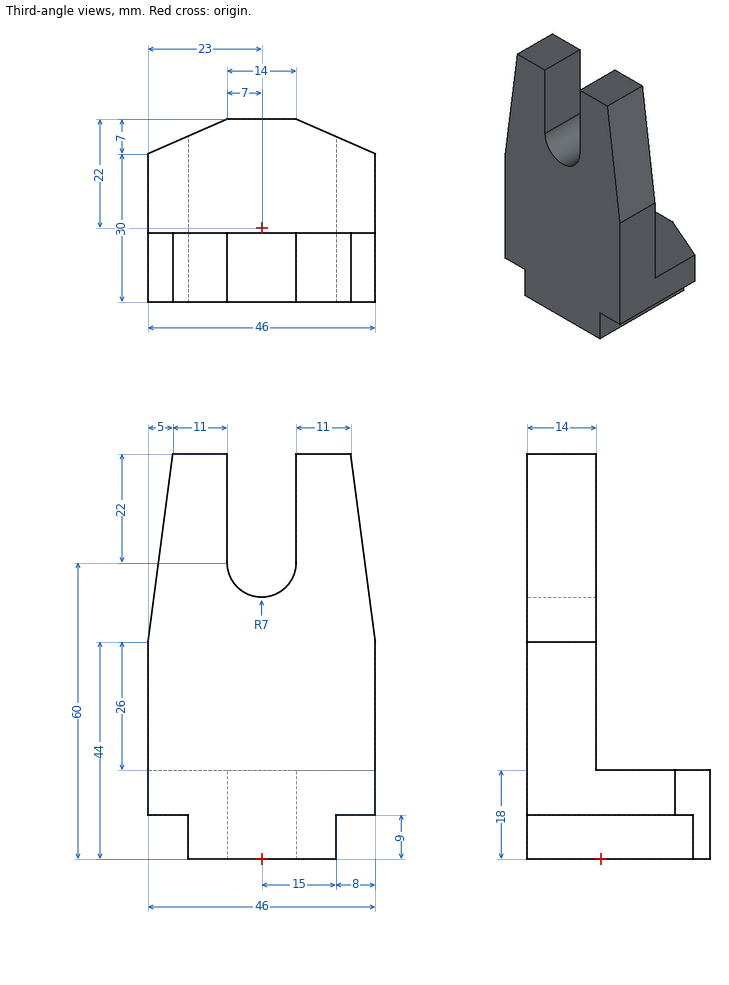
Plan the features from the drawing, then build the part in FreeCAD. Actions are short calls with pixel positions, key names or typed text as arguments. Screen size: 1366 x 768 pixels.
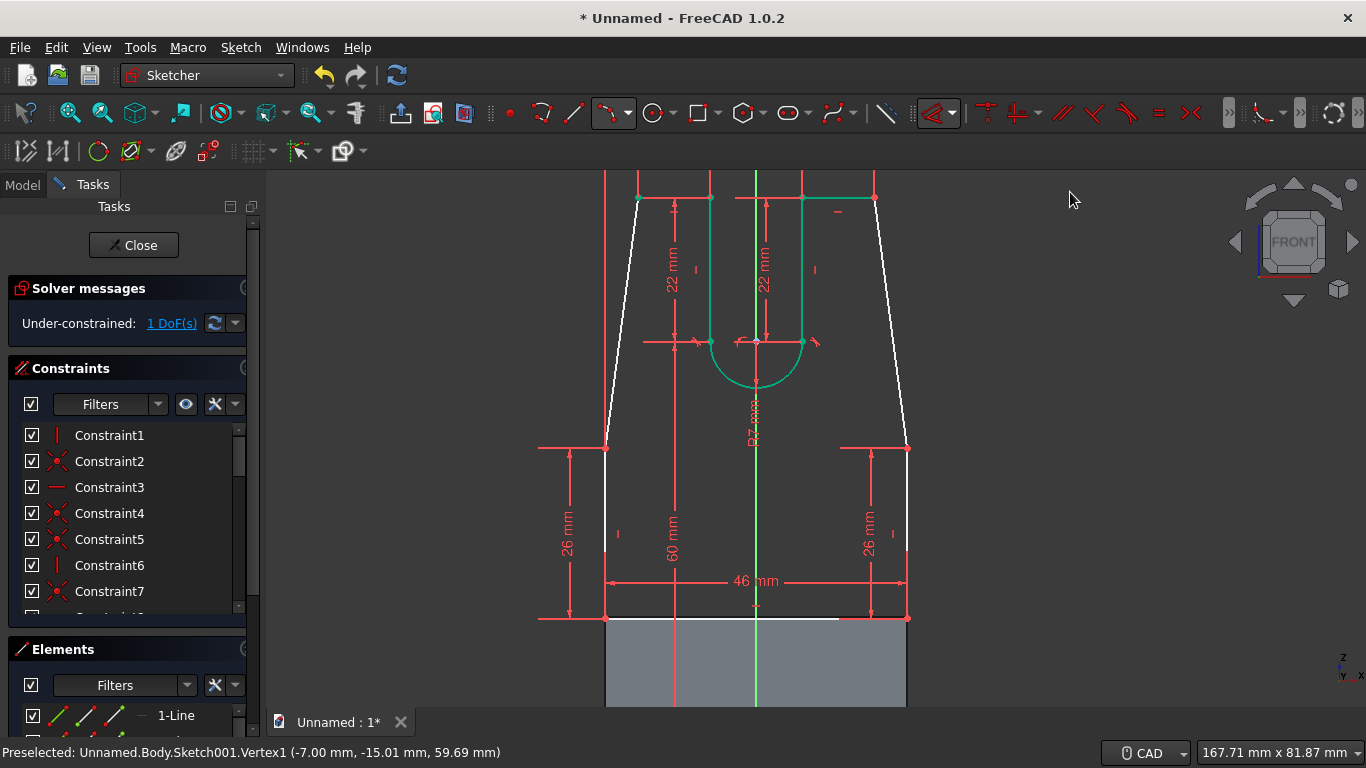
click(605, 448)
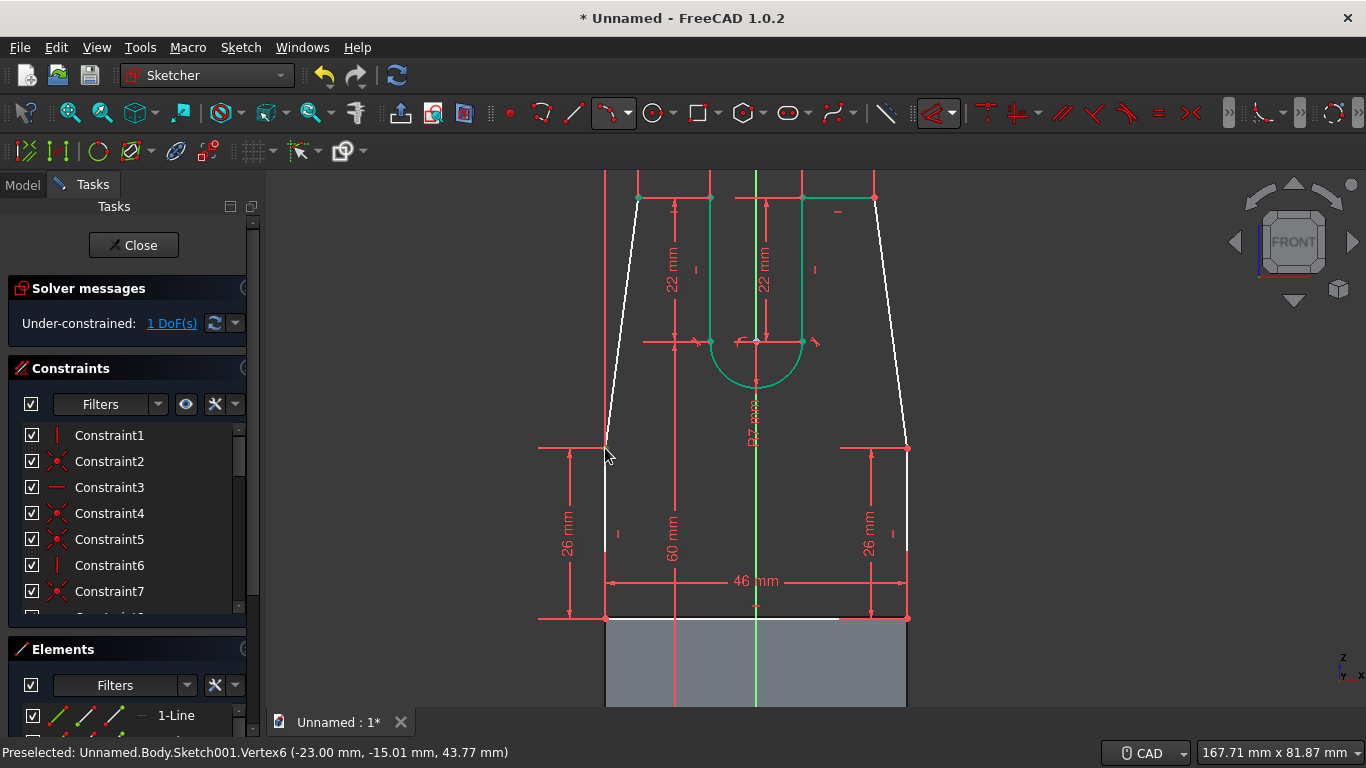
click(954, 114)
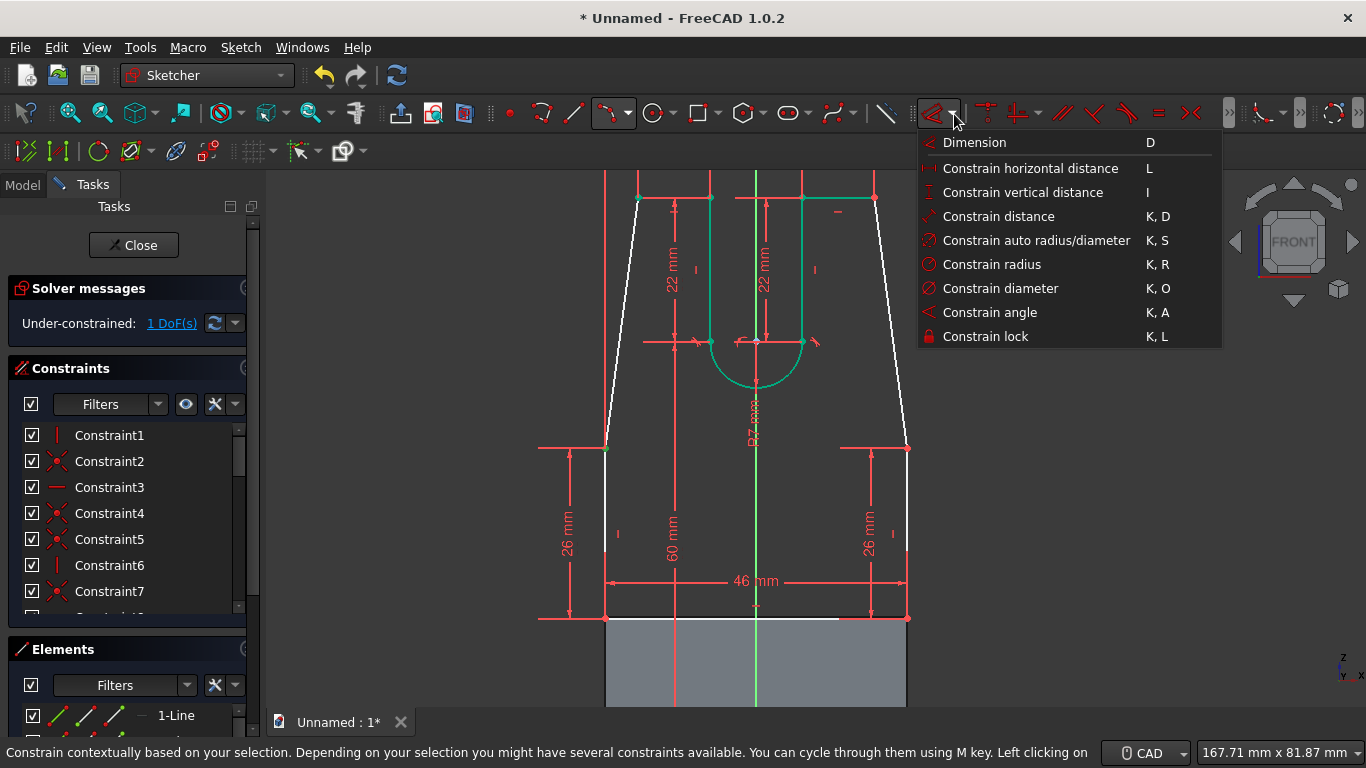
click(1070, 192)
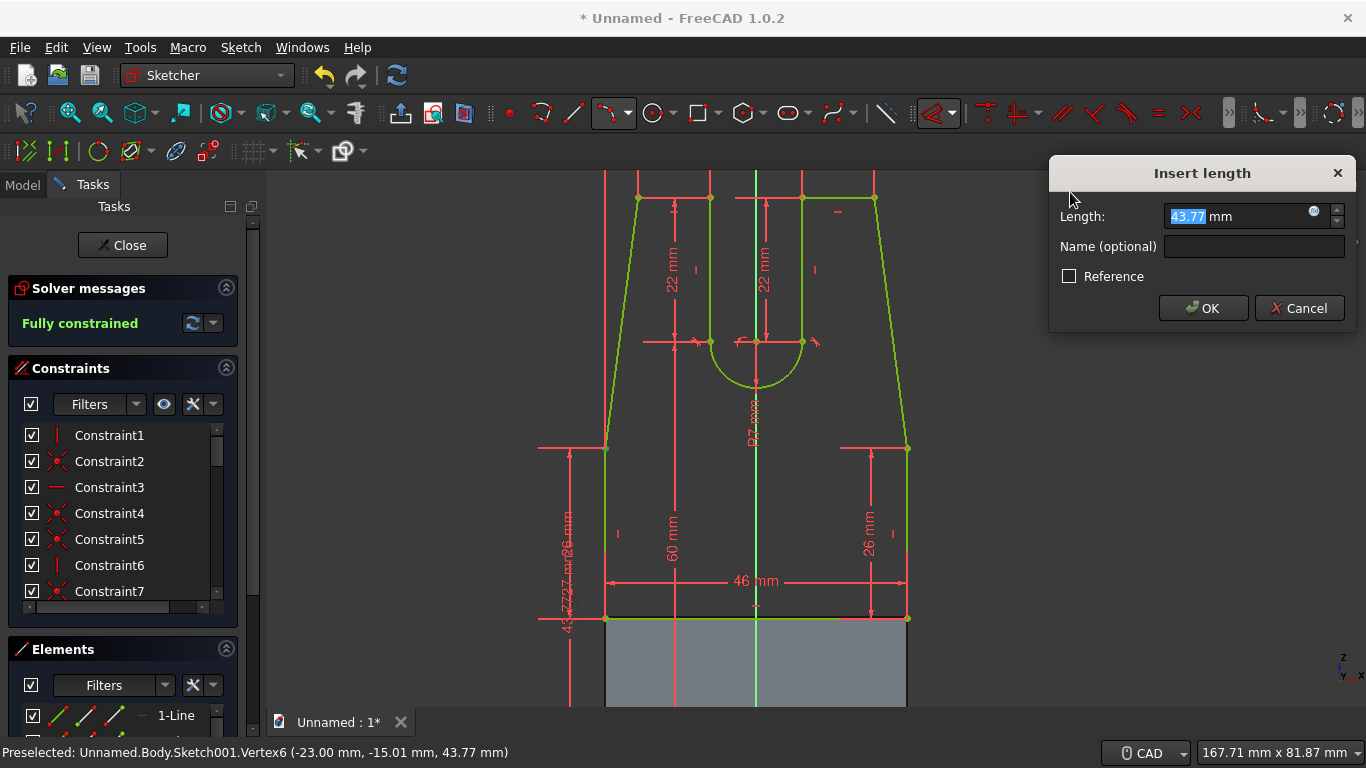
text(44)
key(Return)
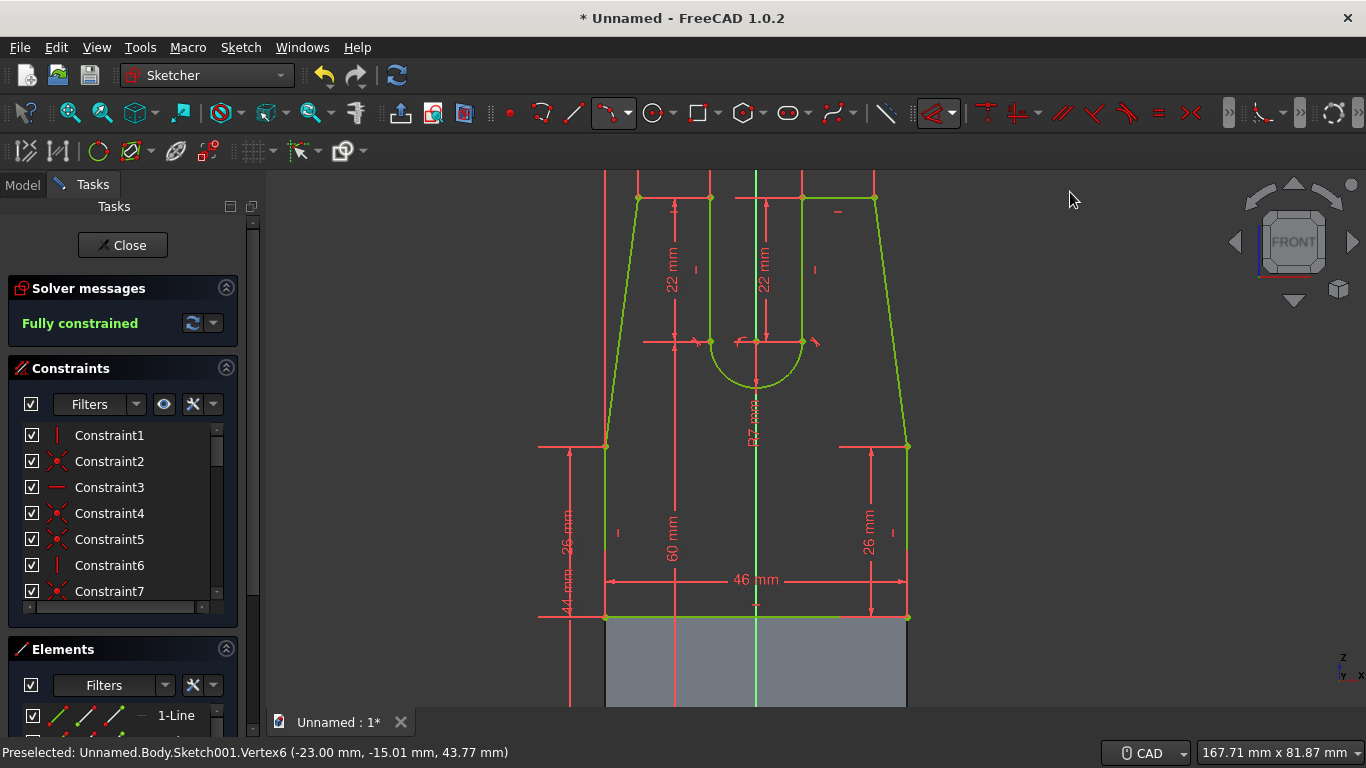
click(123, 245)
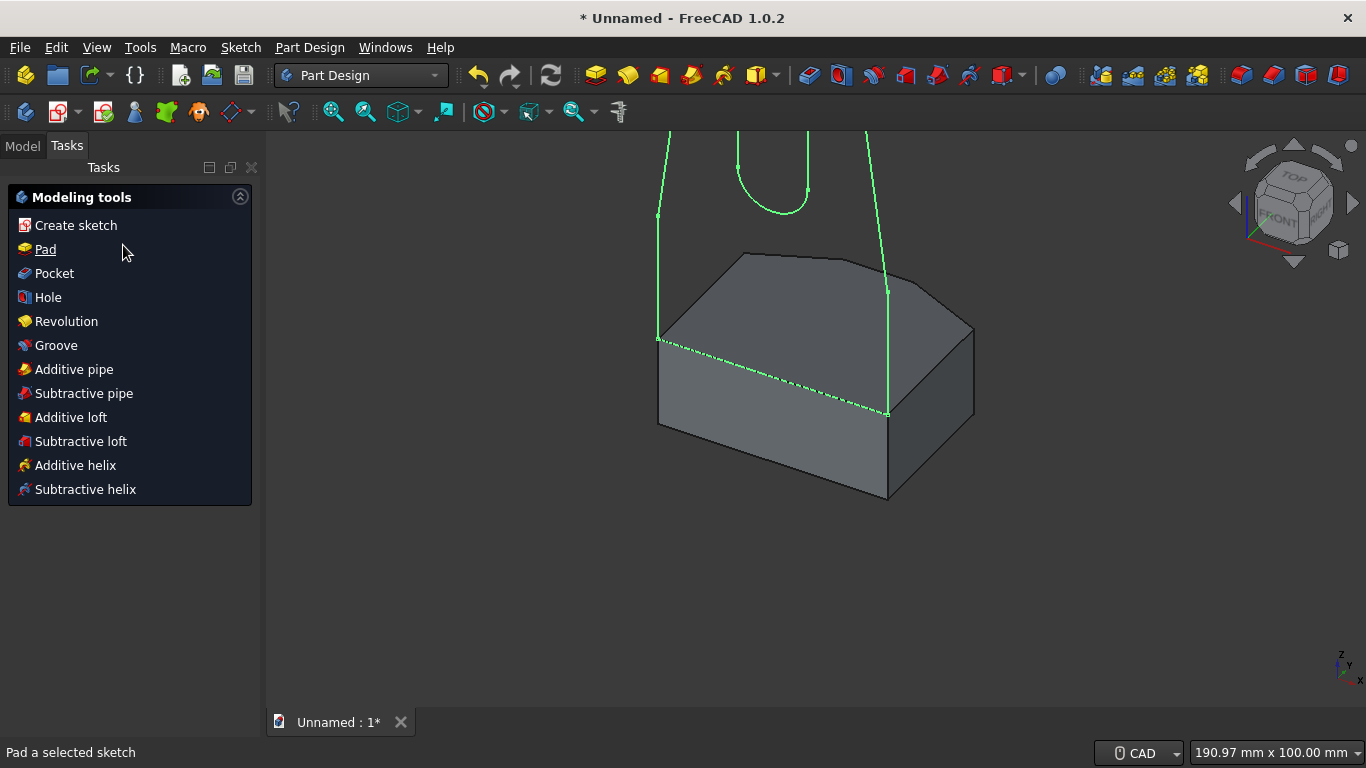
click(596, 76)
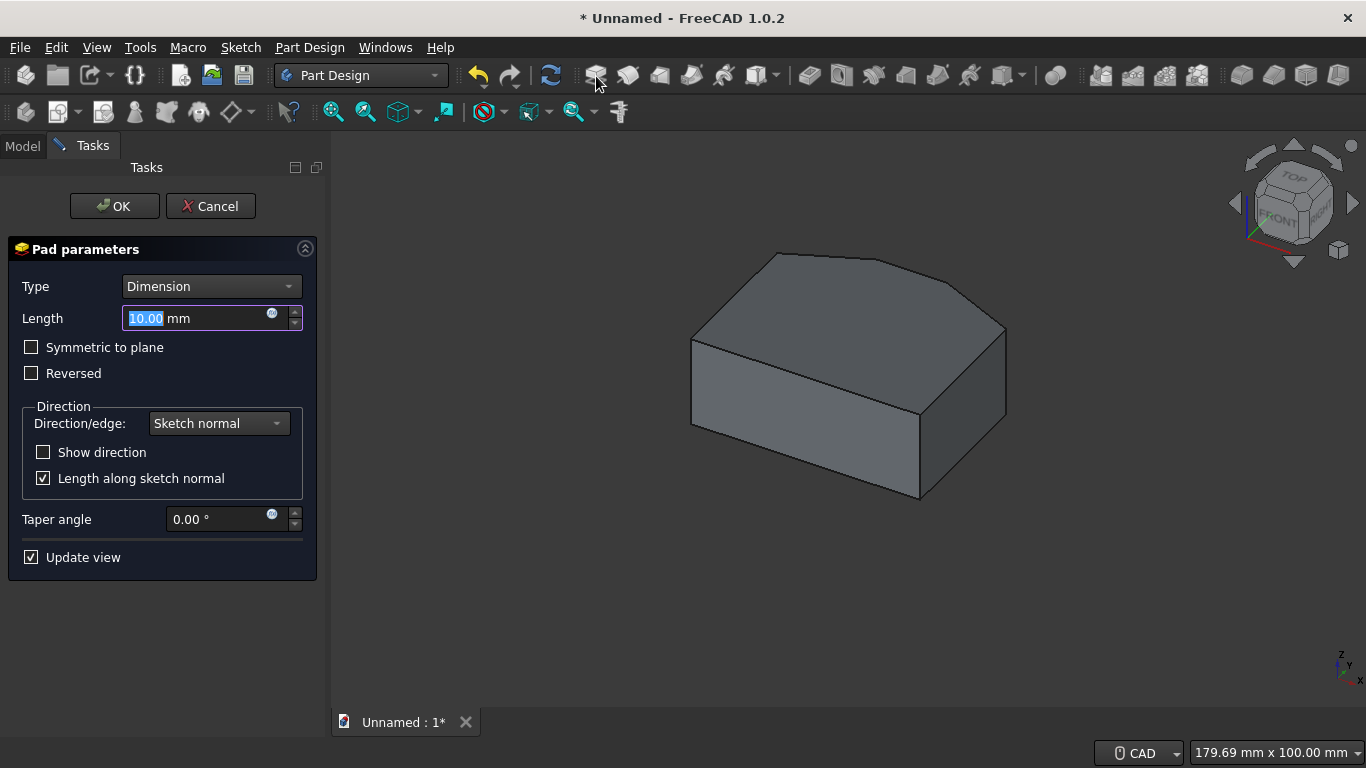
text(14)
key(Tab)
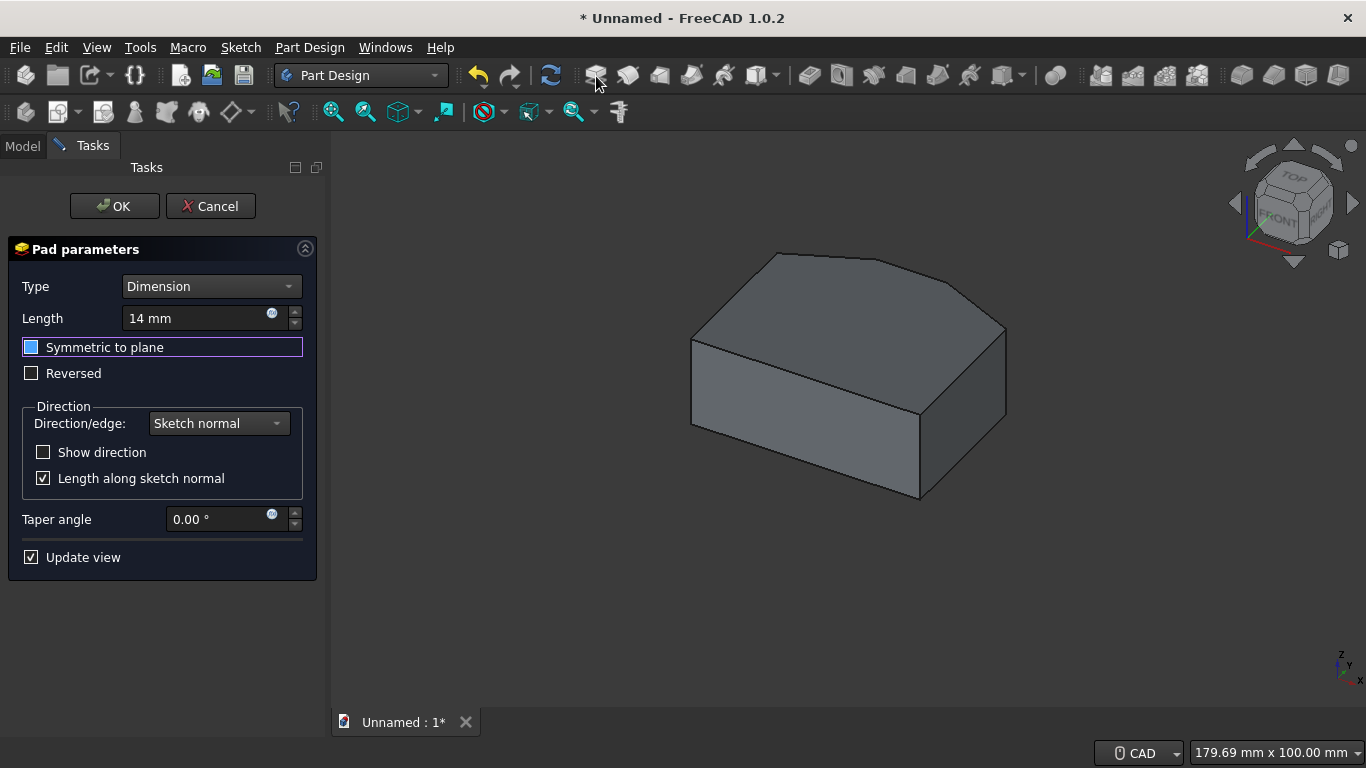
click(30, 373)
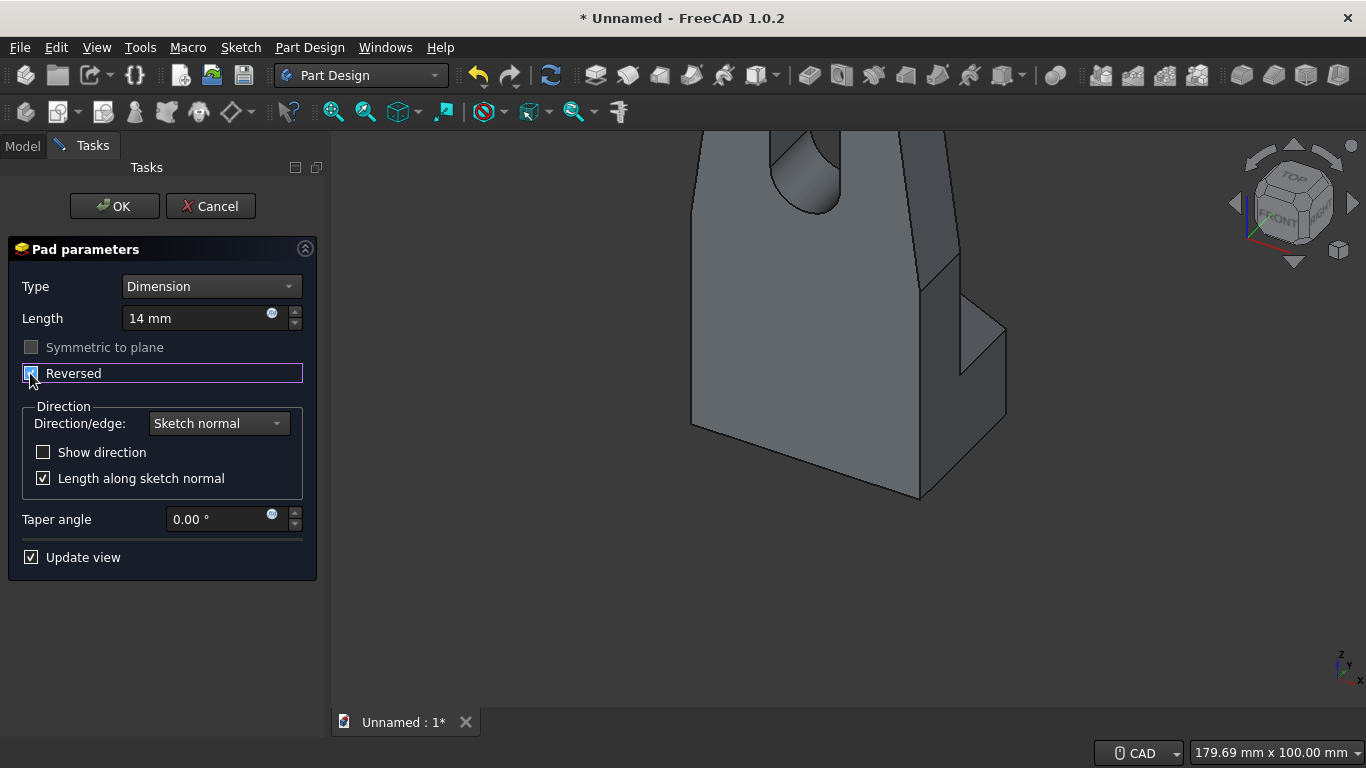
click(115, 206)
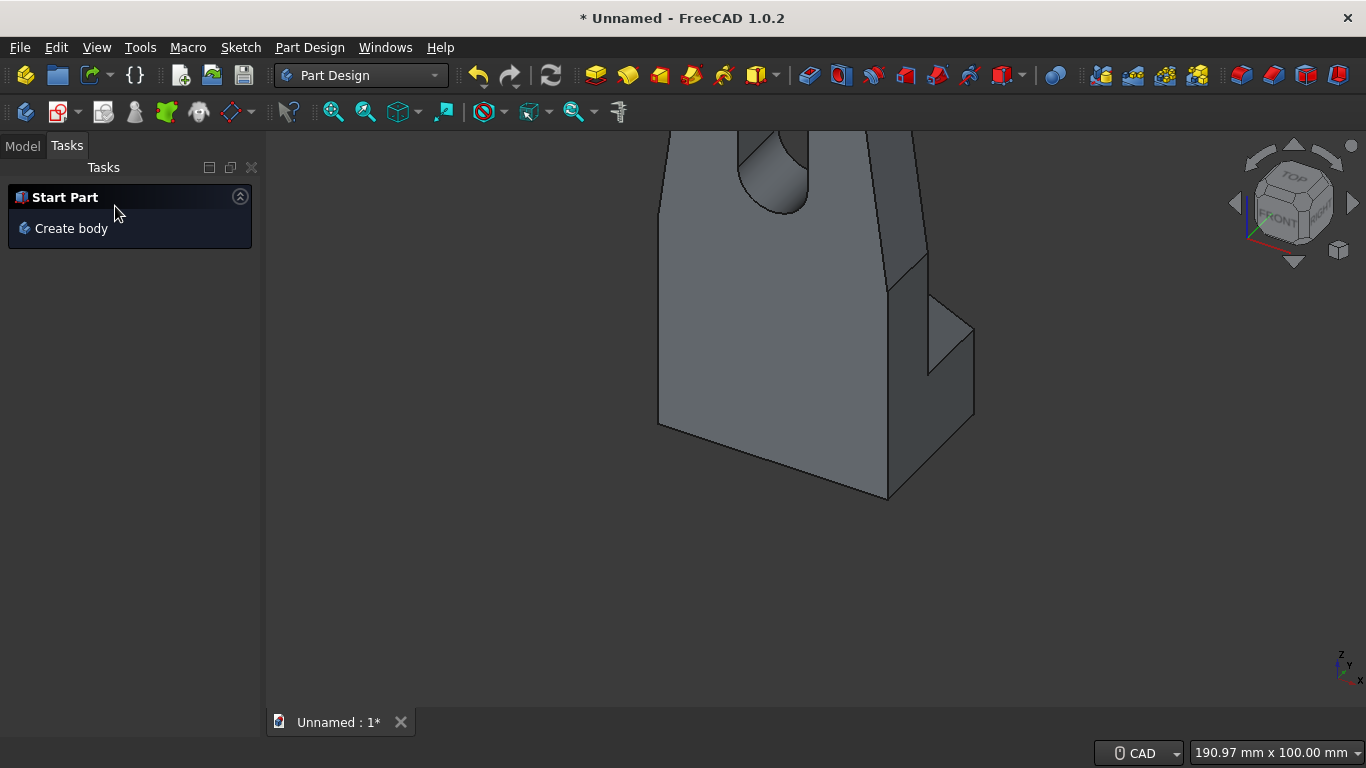
click(334, 112)